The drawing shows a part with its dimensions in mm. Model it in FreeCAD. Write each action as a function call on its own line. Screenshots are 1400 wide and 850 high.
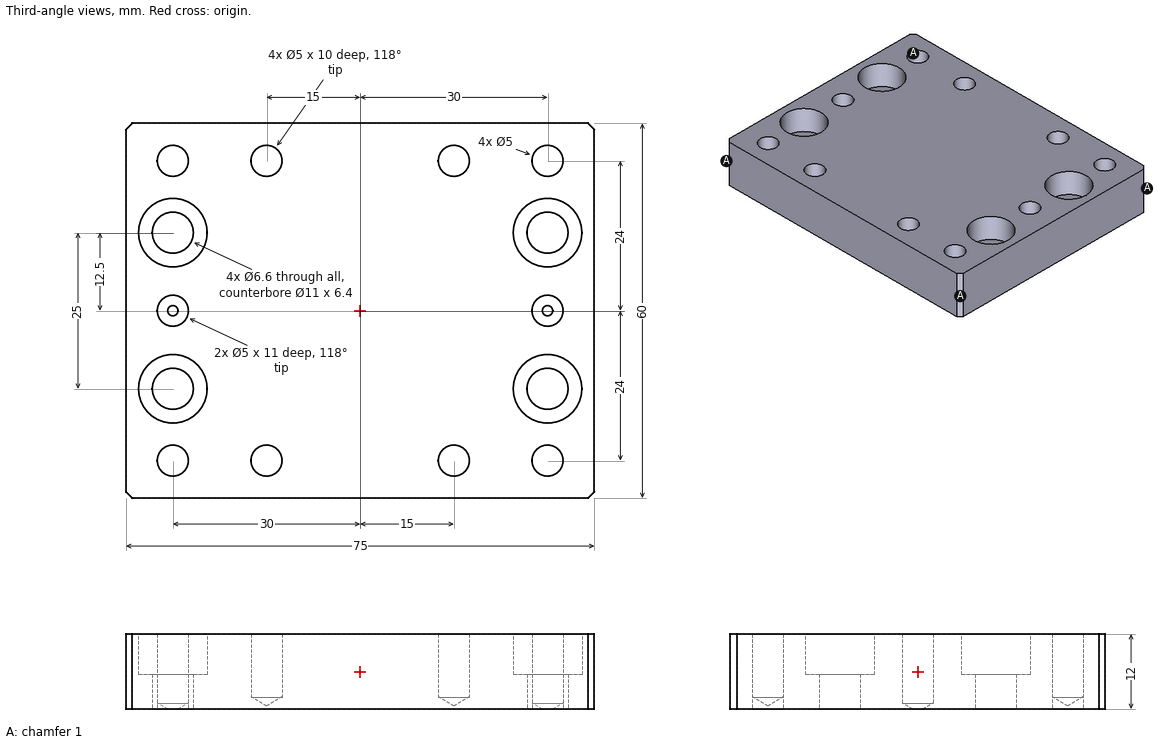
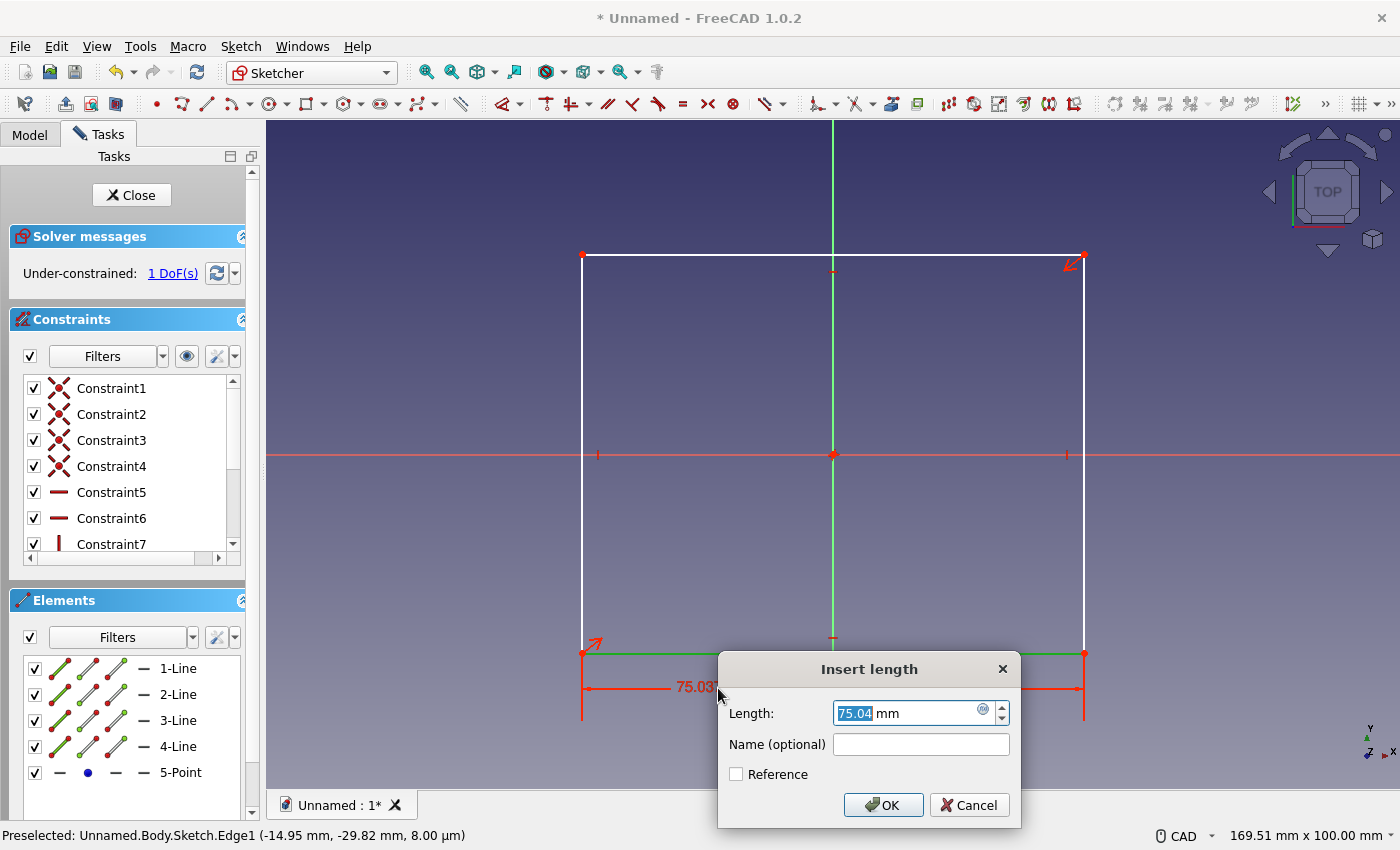
text(75)
key(Return)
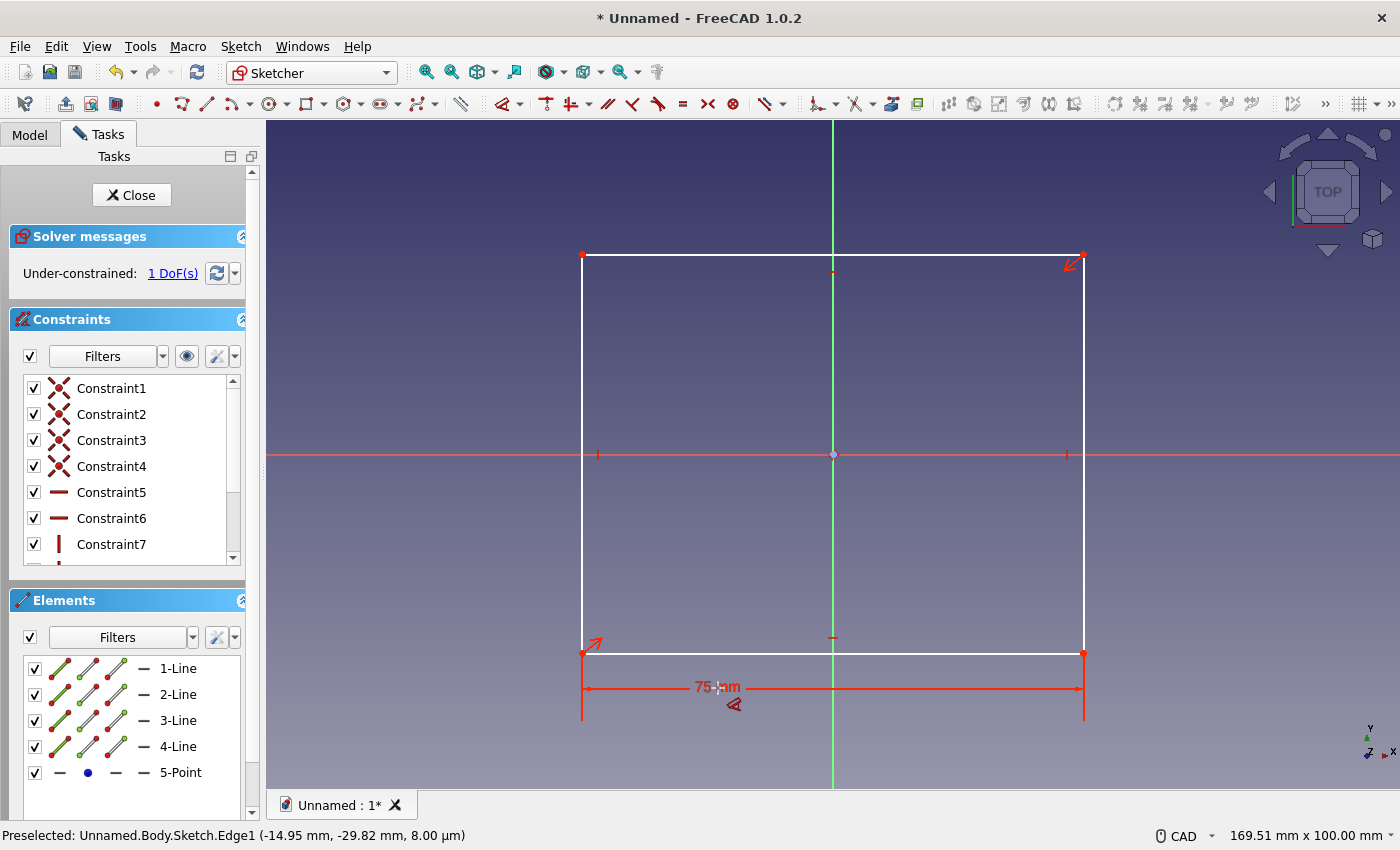
click(1084, 534)
click(1118, 363)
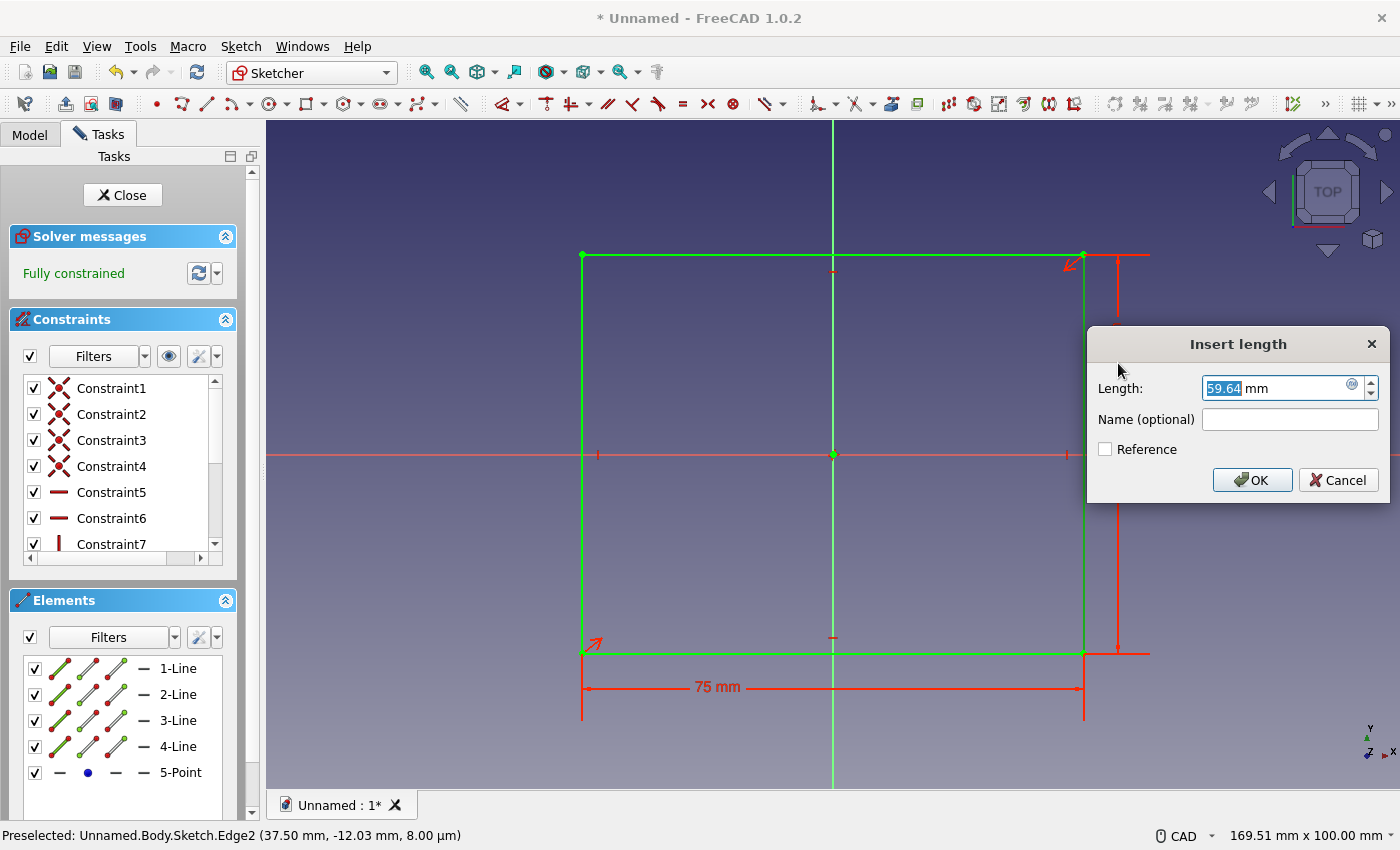
text(60)
key(Return)
key(Escape)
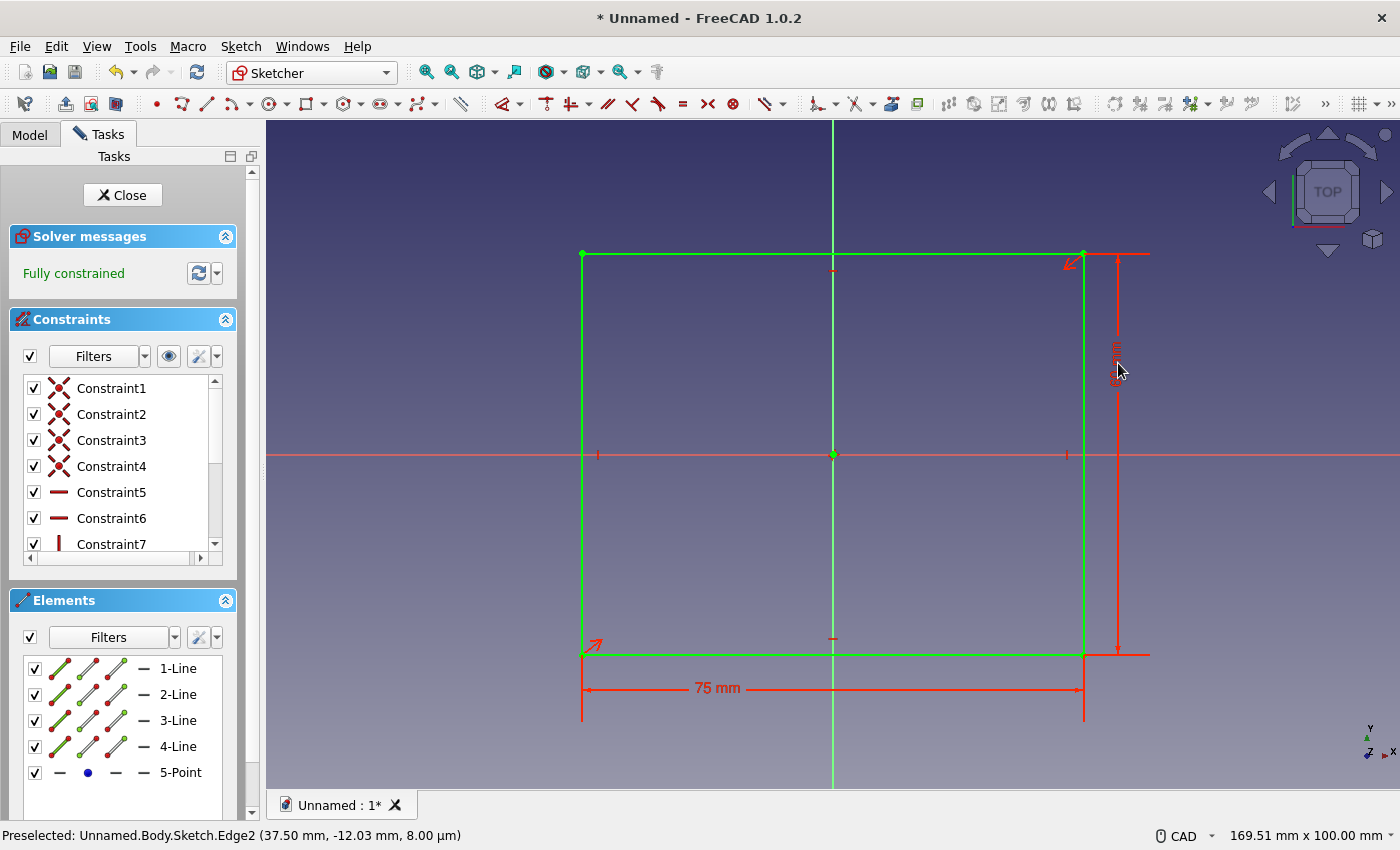
click(123, 195)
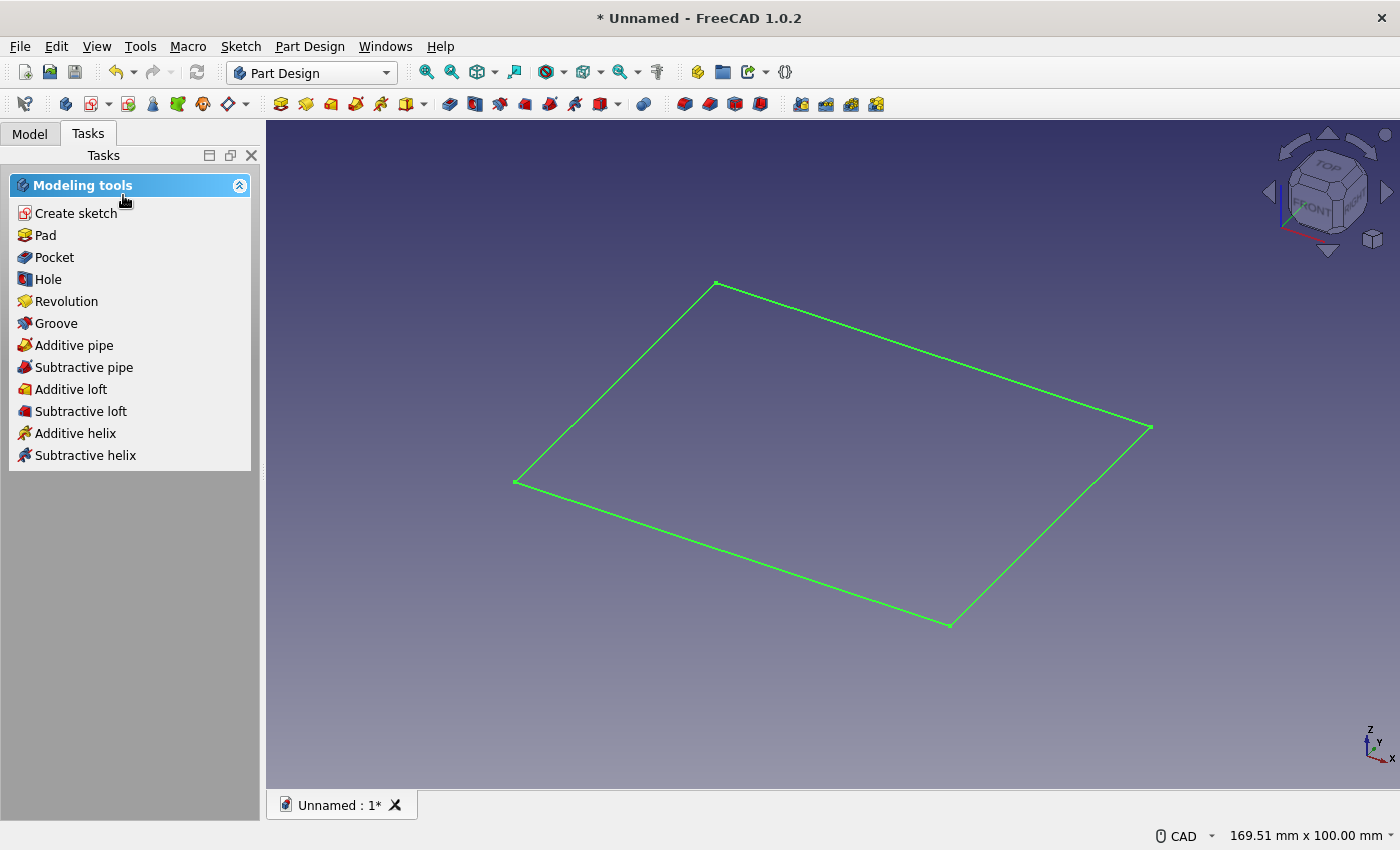
click(281, 104)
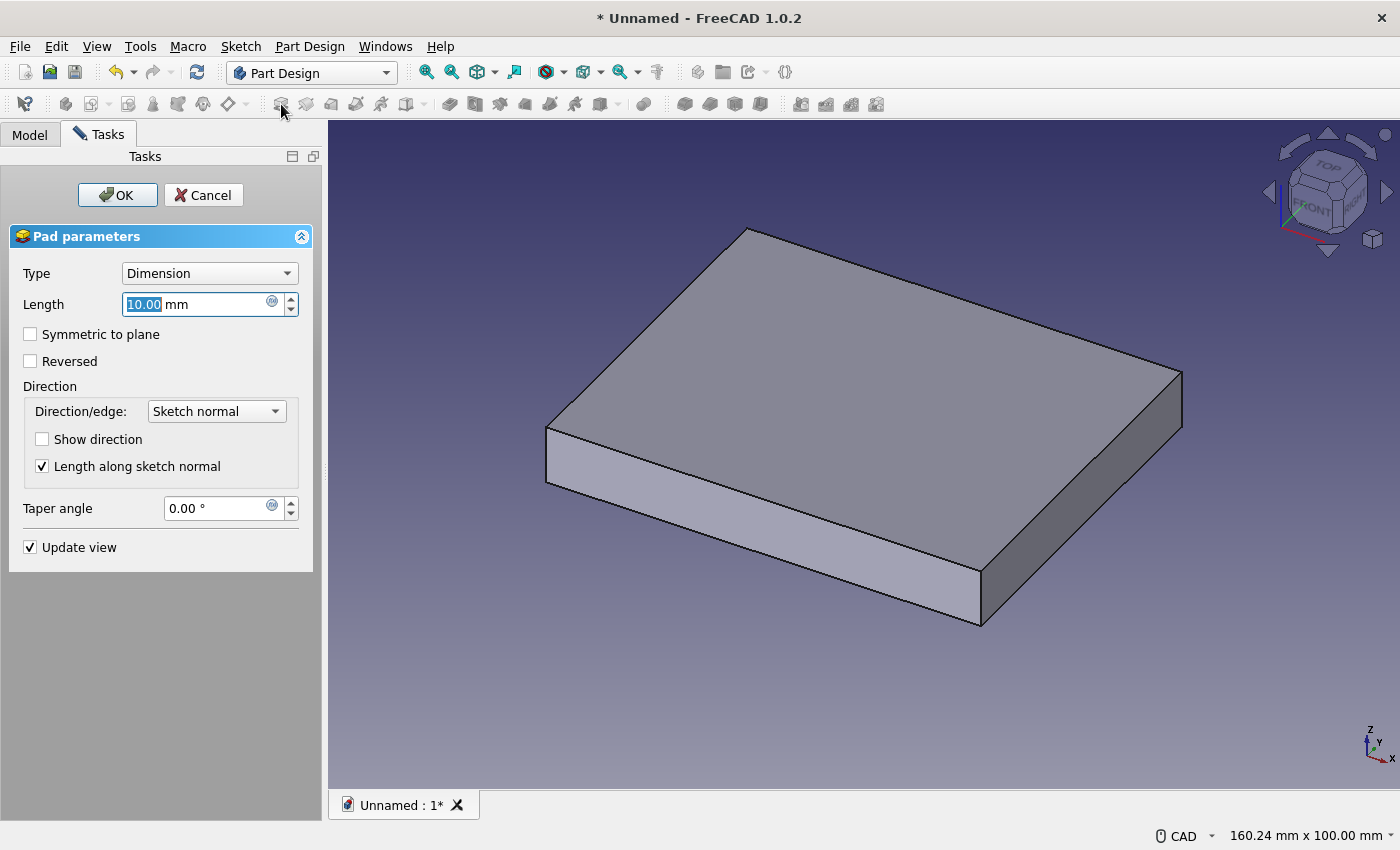
text(12)
key(Tab)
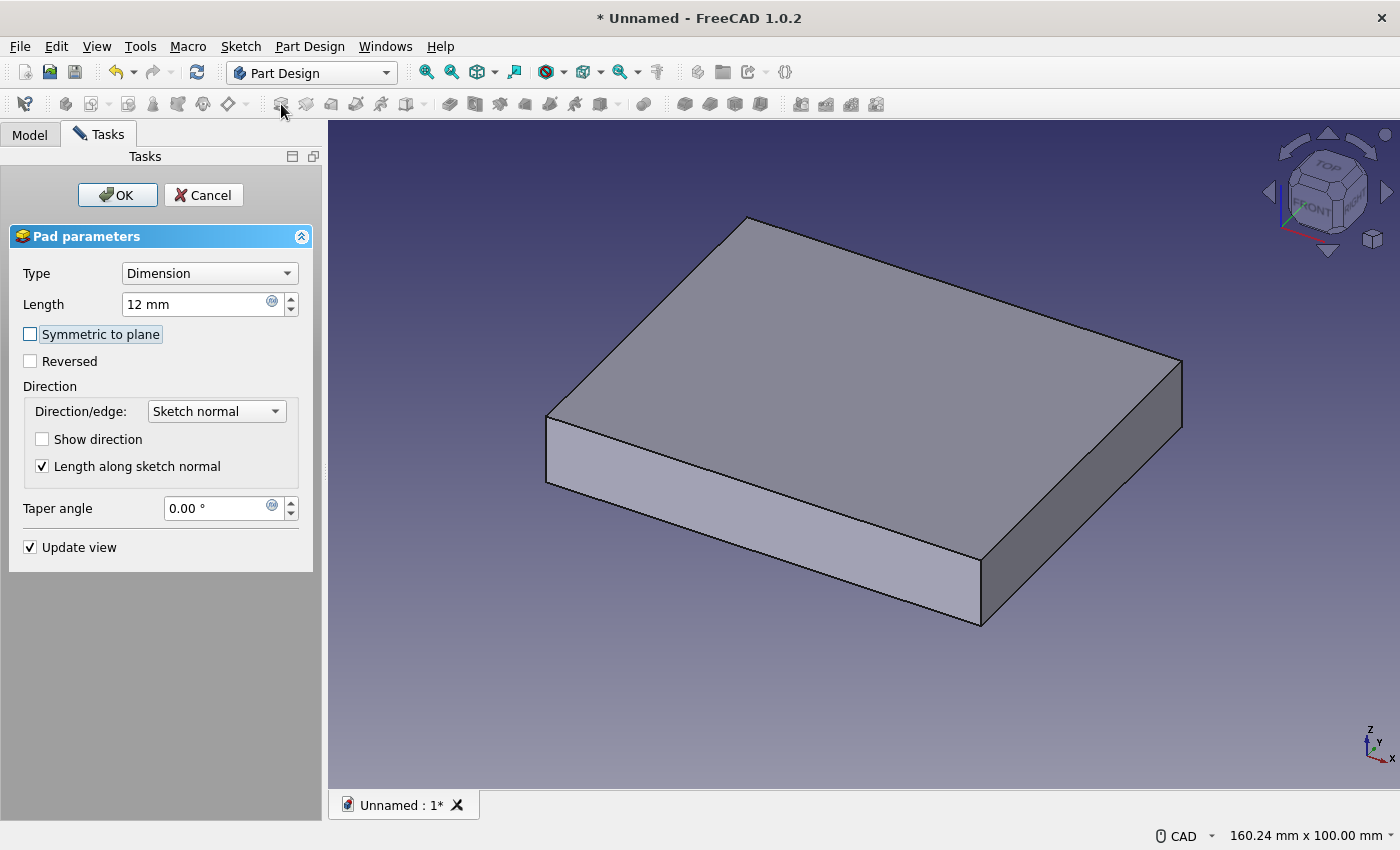
click(31, 334)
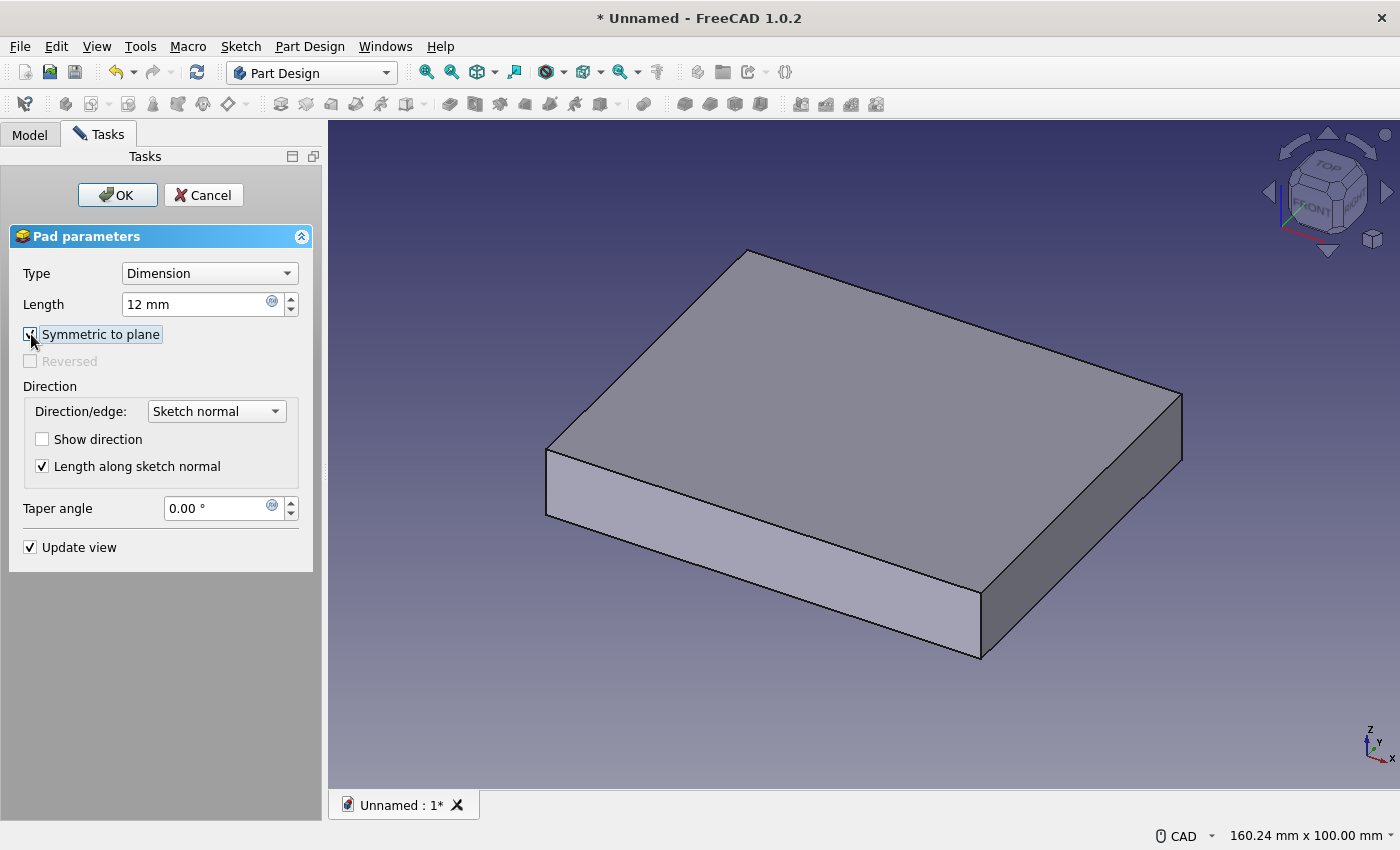
click(118, 195)